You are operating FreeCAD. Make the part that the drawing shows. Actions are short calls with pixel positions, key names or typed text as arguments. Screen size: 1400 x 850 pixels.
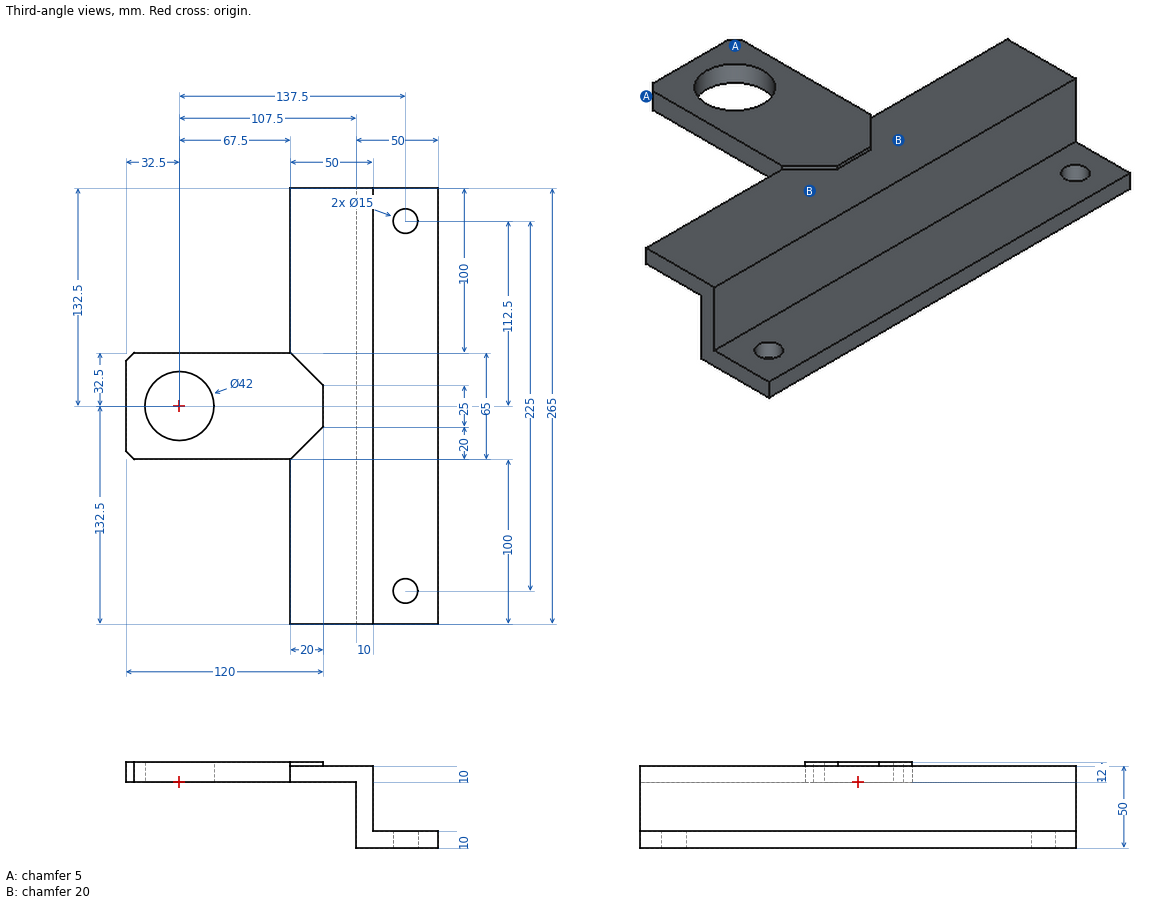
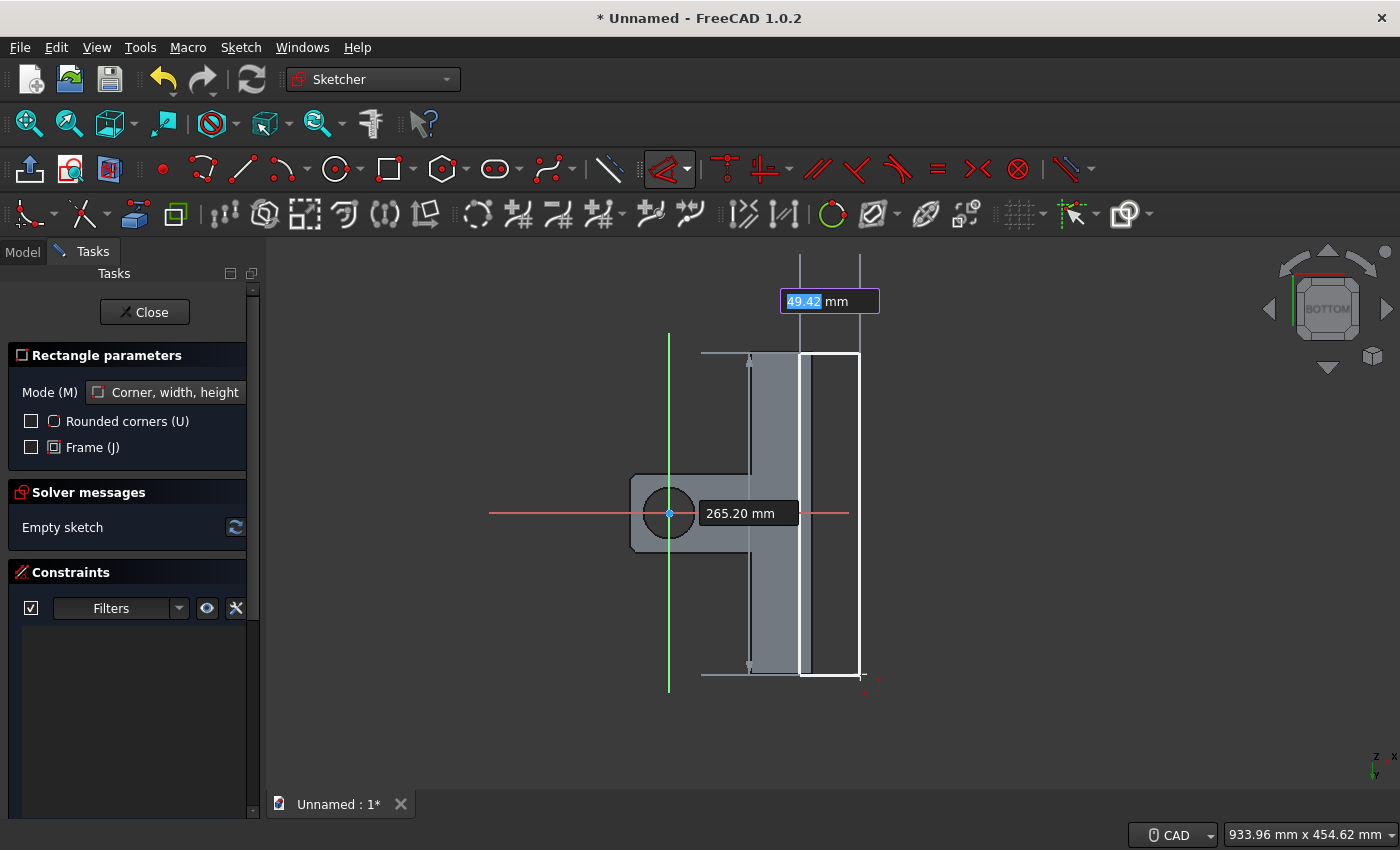
text(50)
key(Tab)
text(265)
key(Return)
key(Escape)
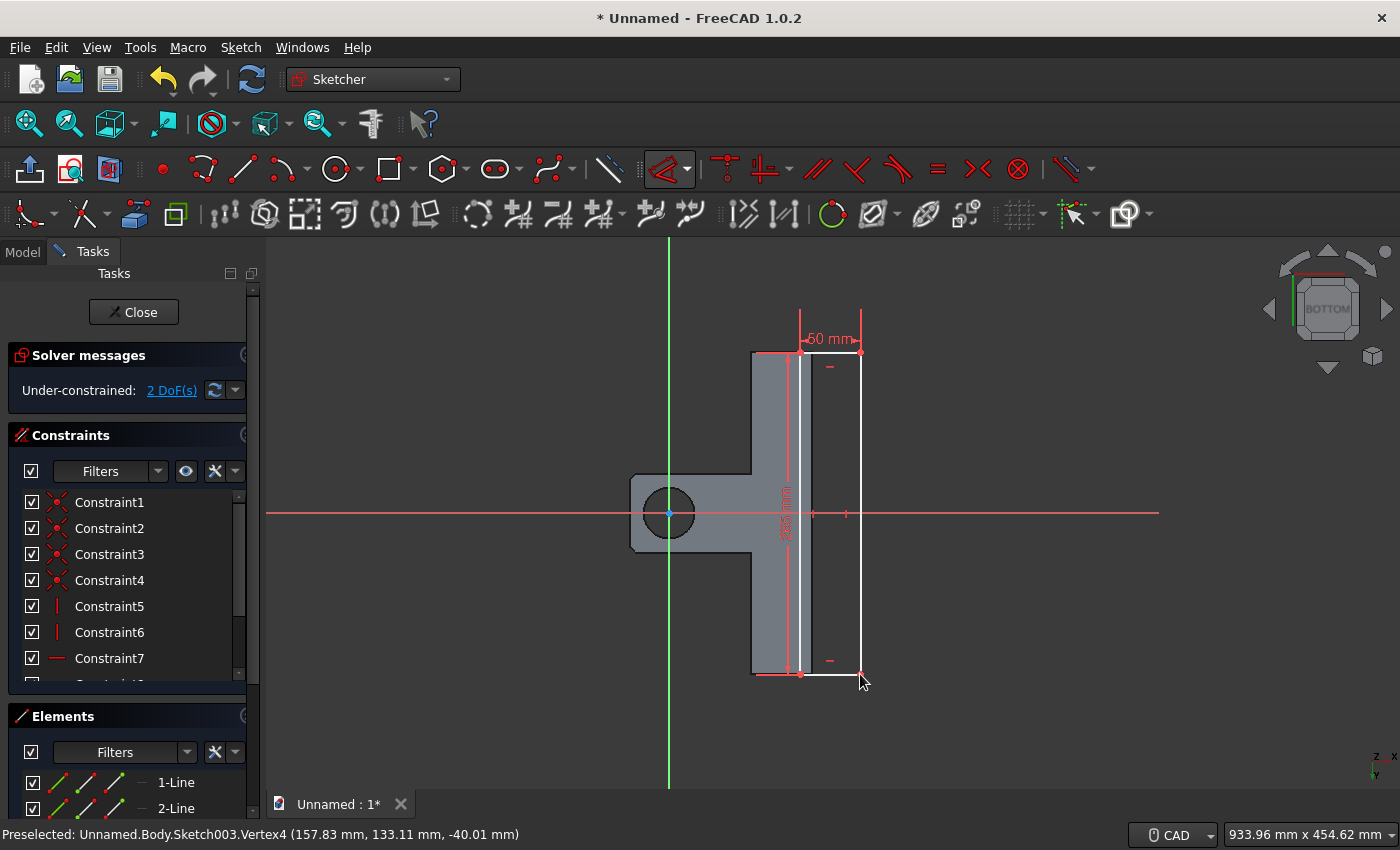
click(800, 353)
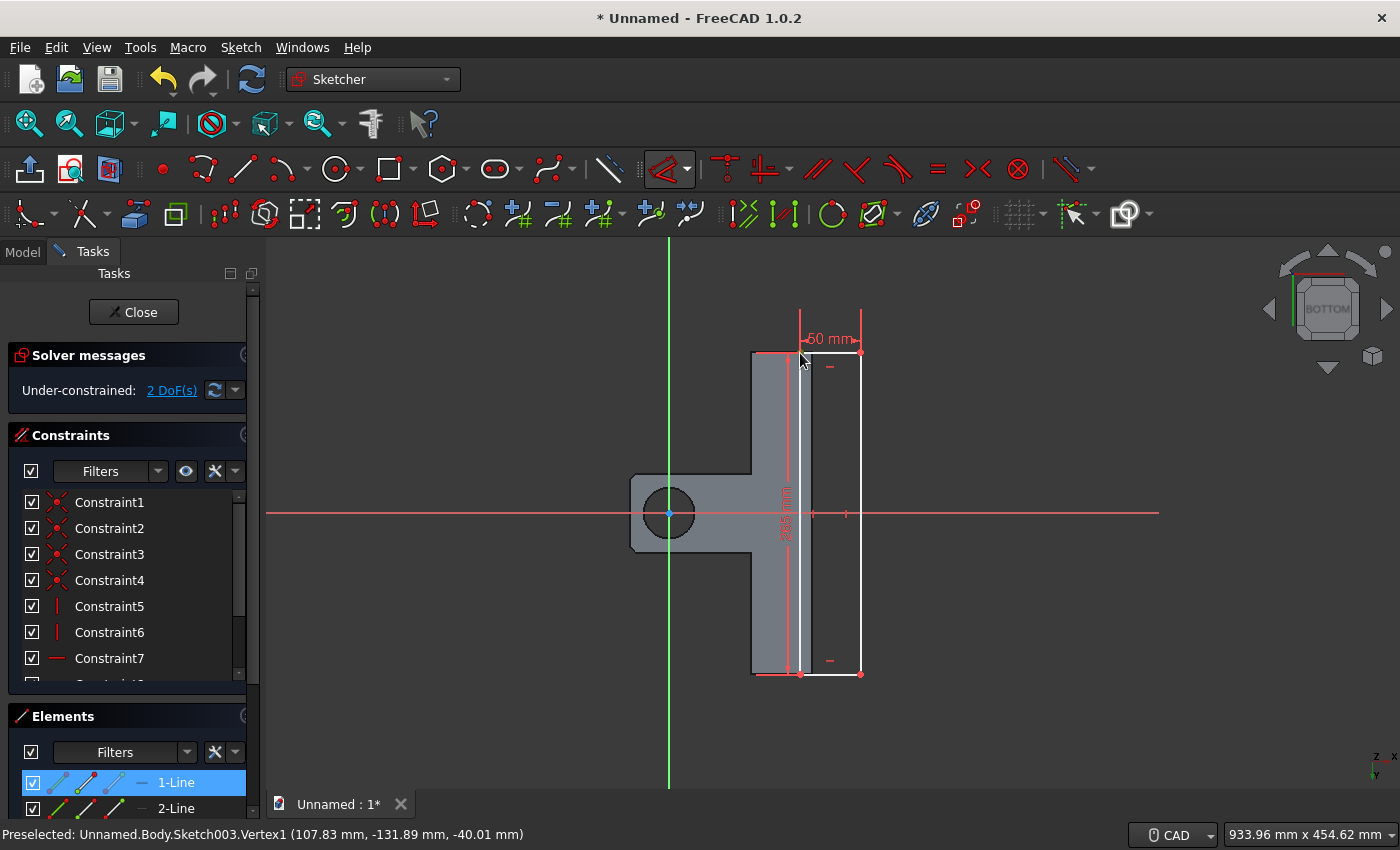
key(l)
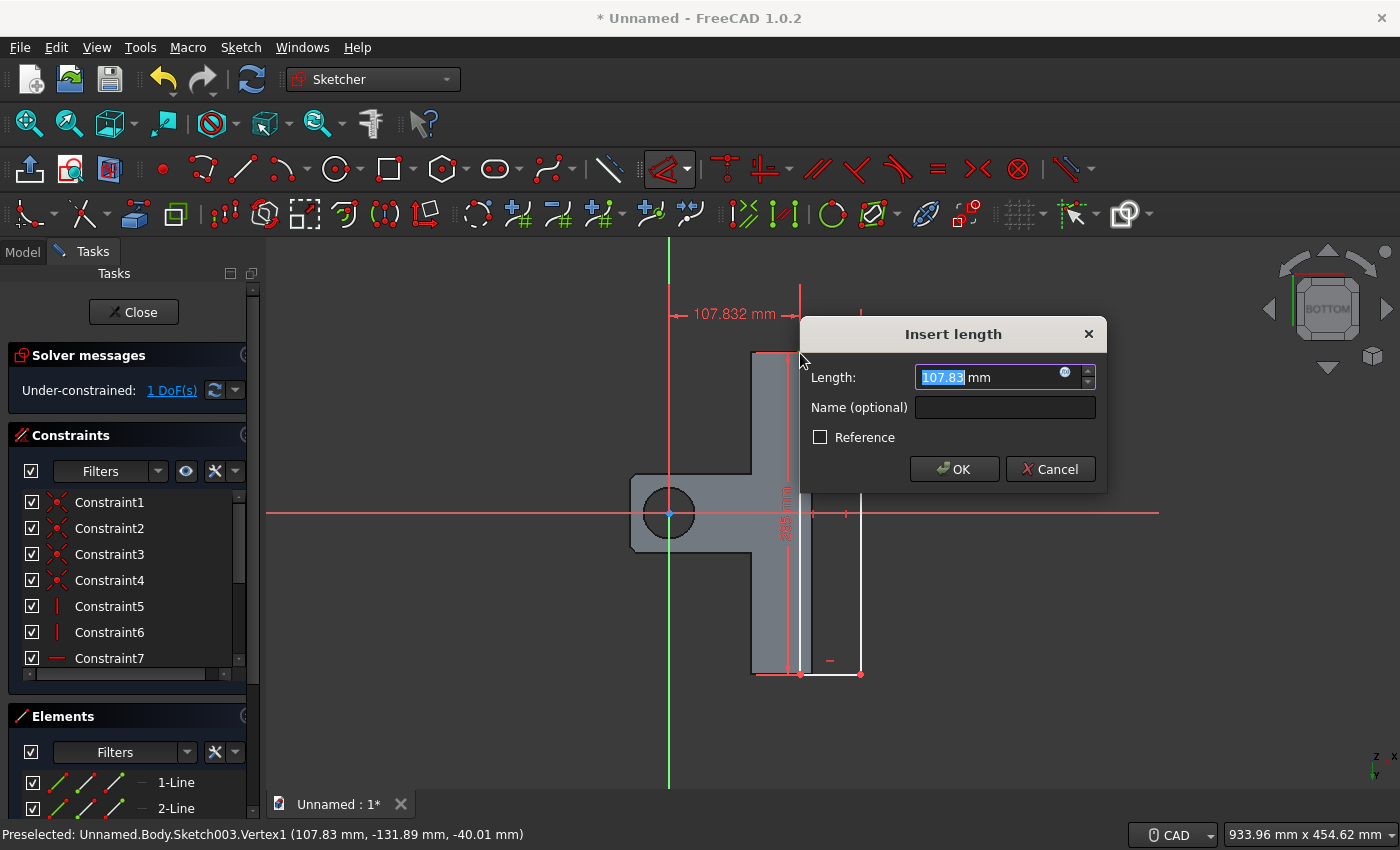
text(107.5)
key(Return)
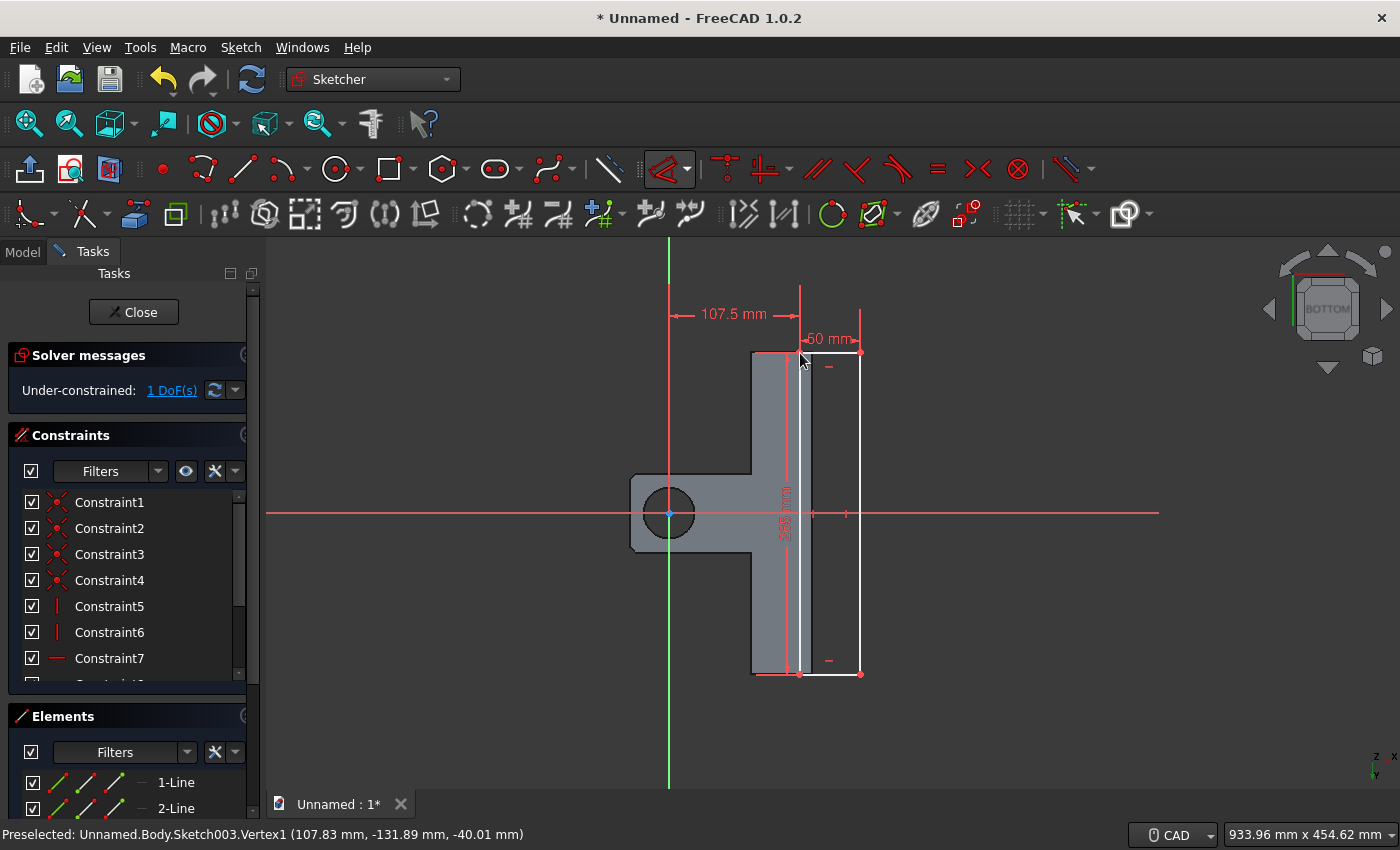
click(800, 353)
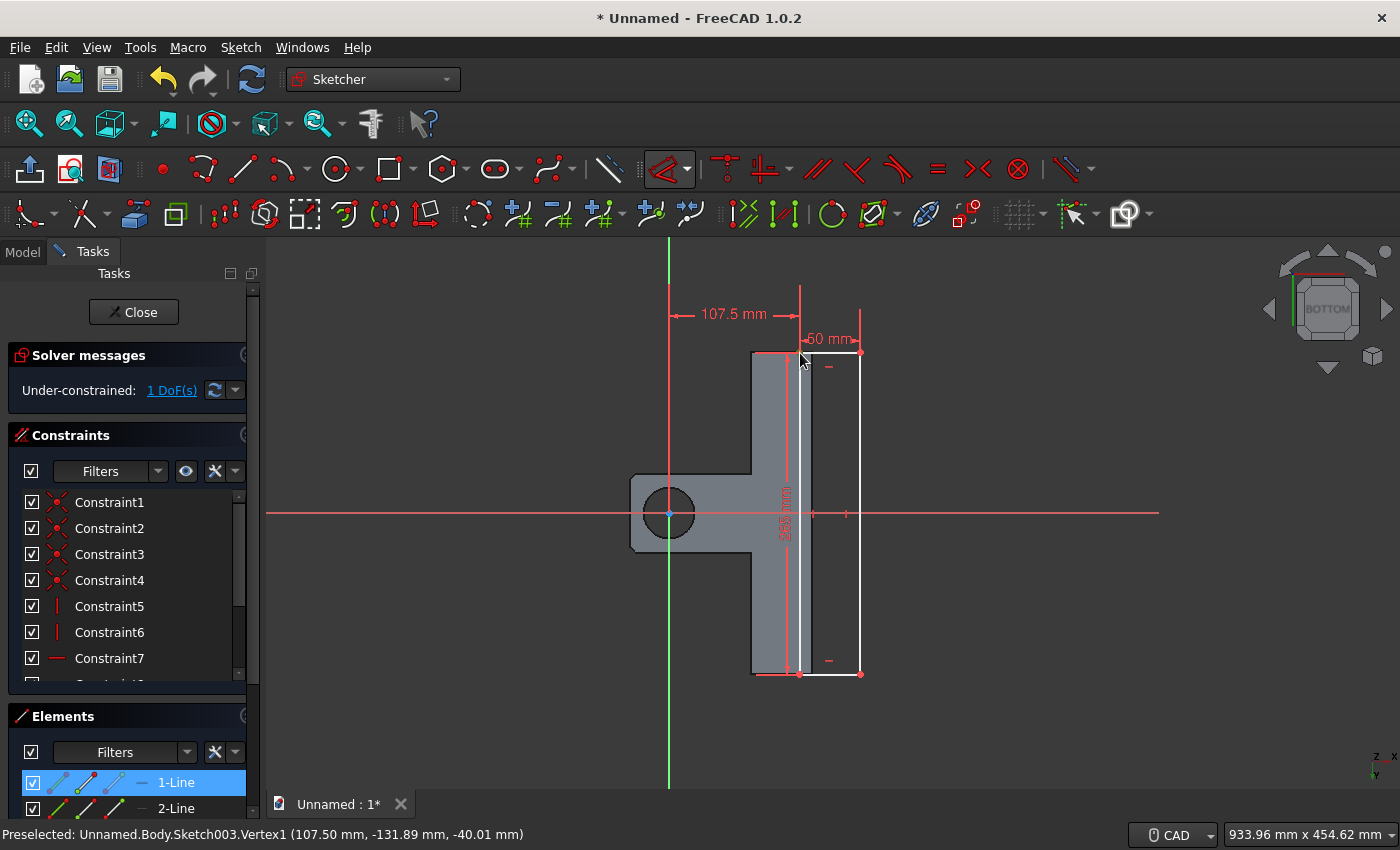
key(i)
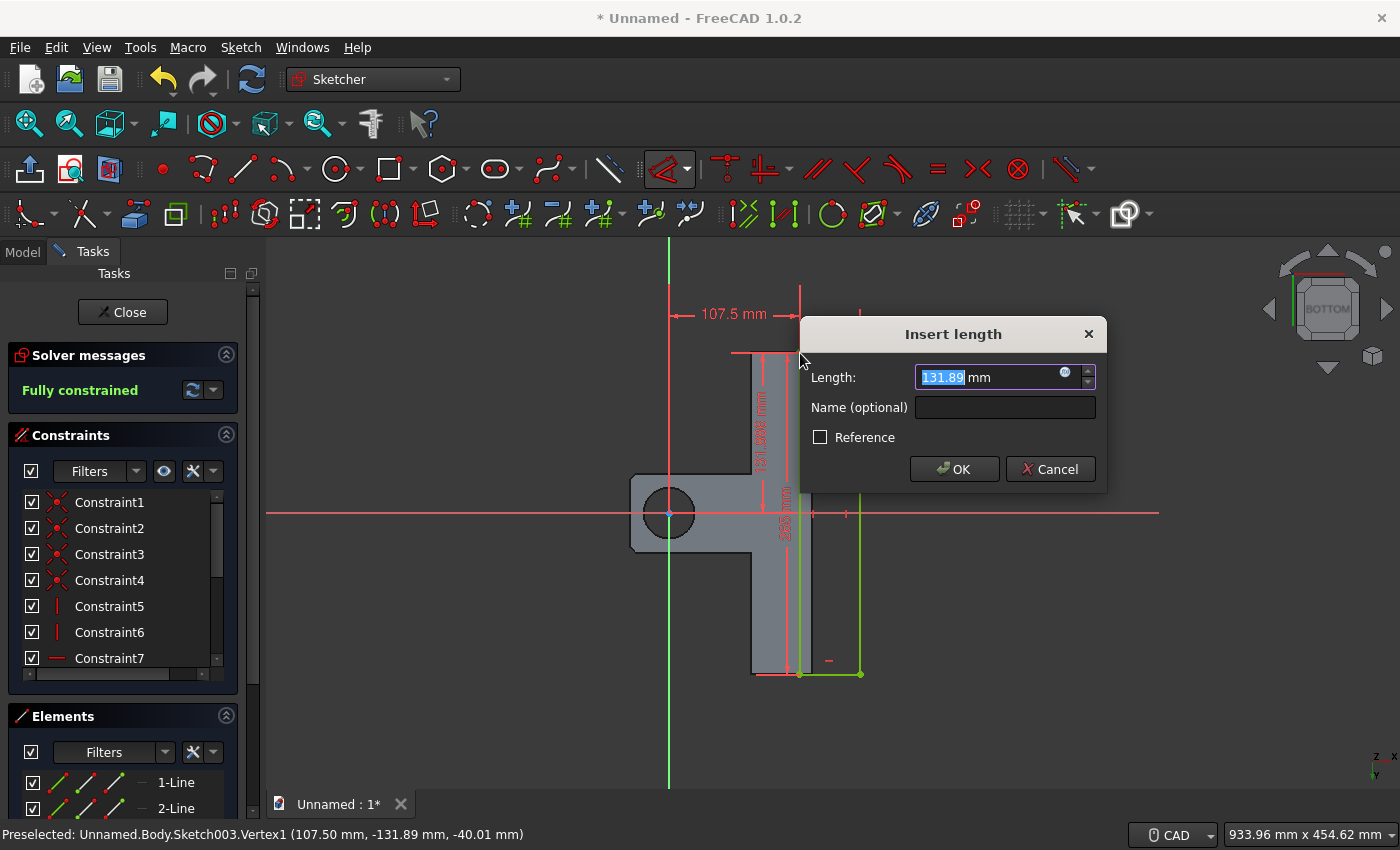
text(132.5)
key(Return)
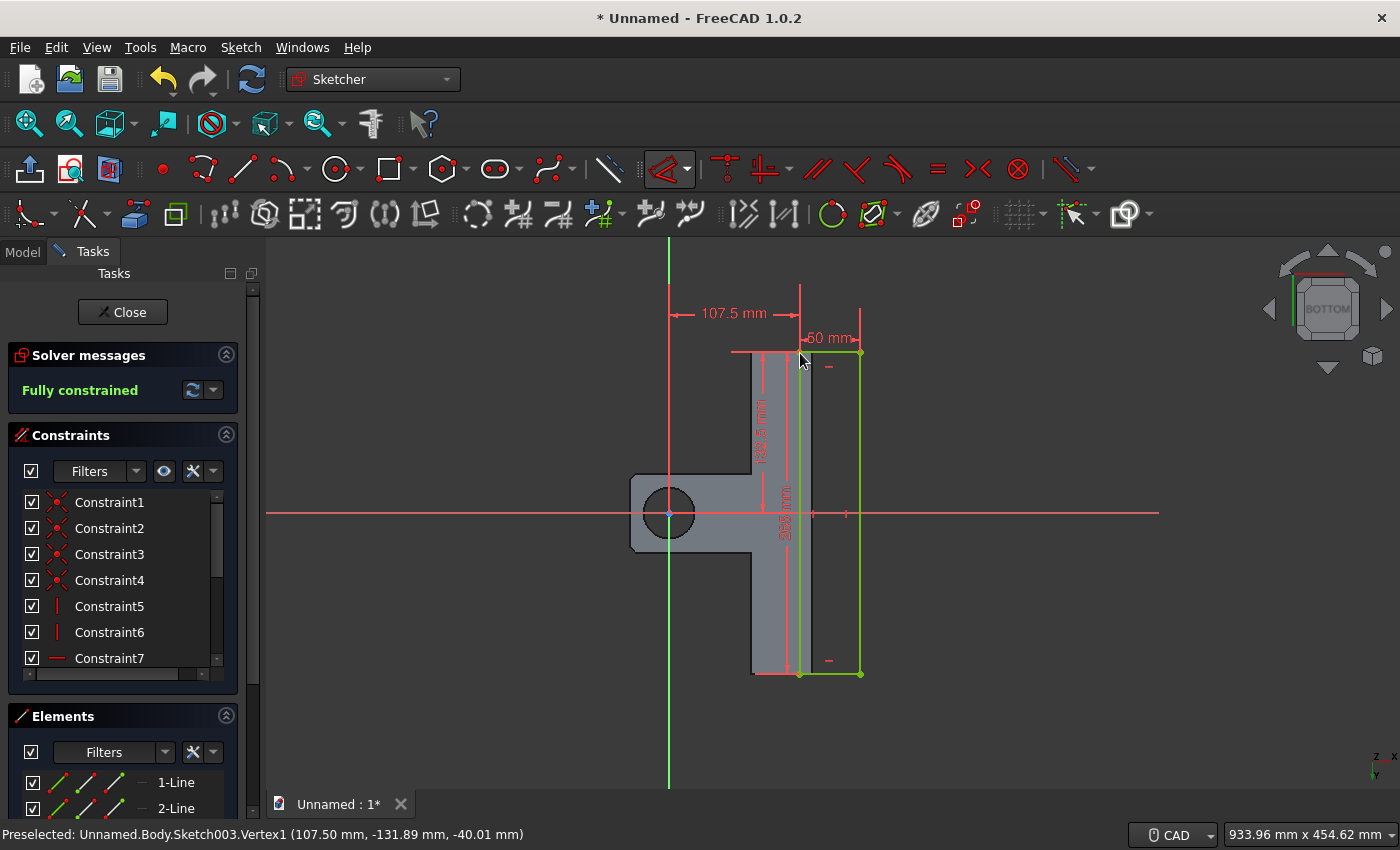
click(123, 312)